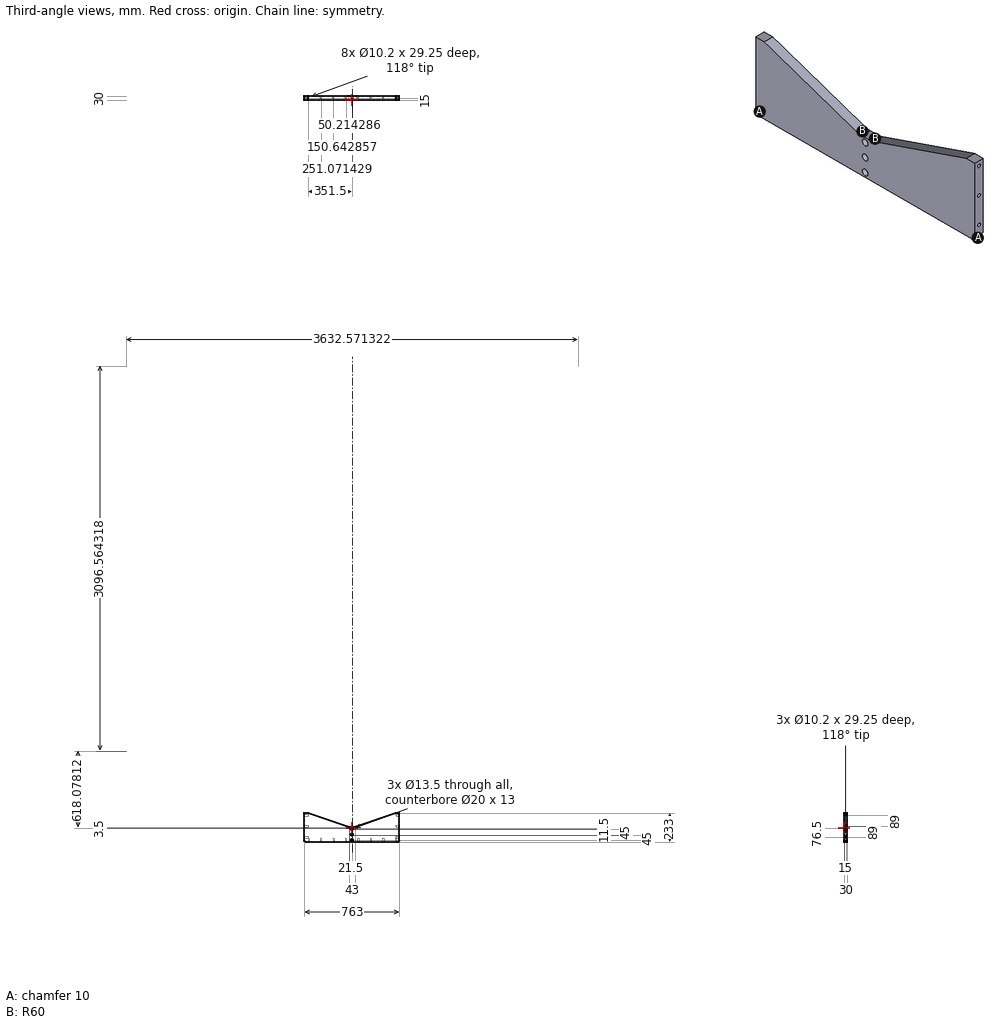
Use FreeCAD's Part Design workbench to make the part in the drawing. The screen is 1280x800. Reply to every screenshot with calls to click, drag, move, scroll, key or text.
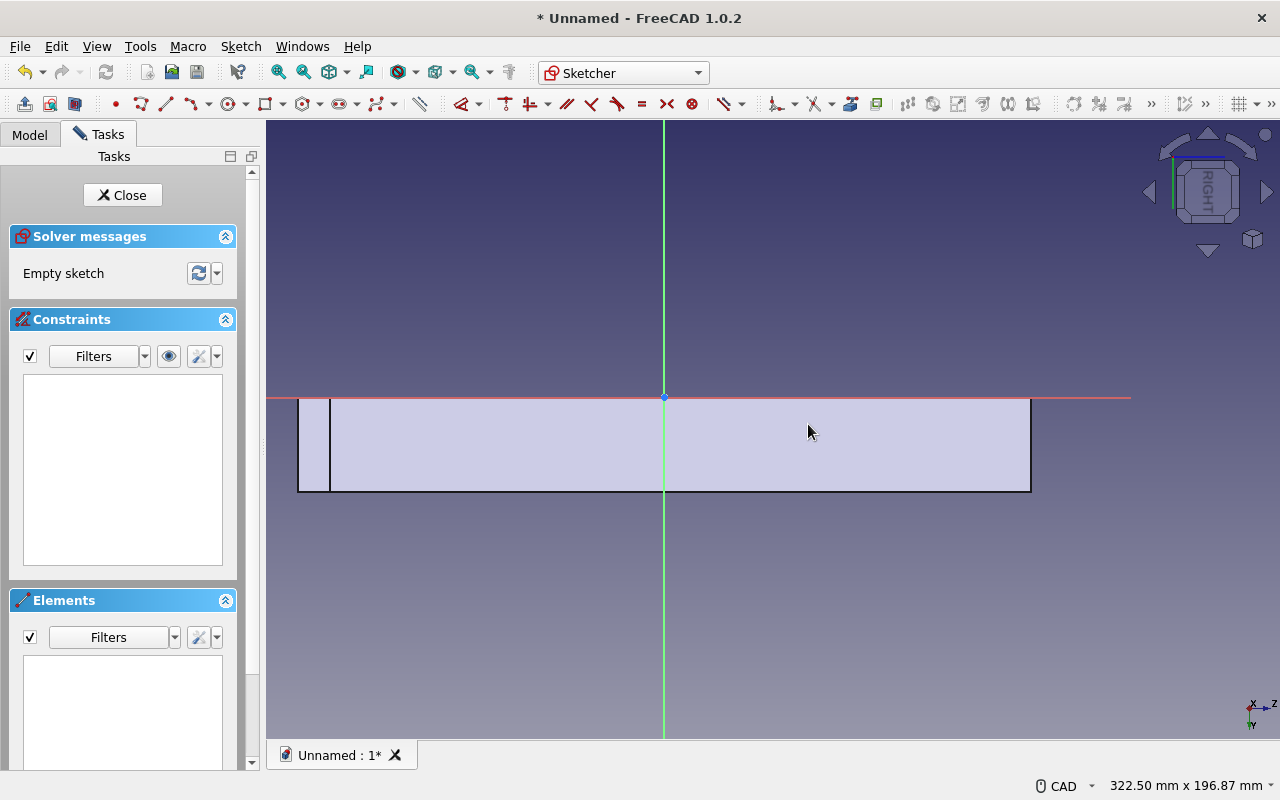
key(g)
key(c)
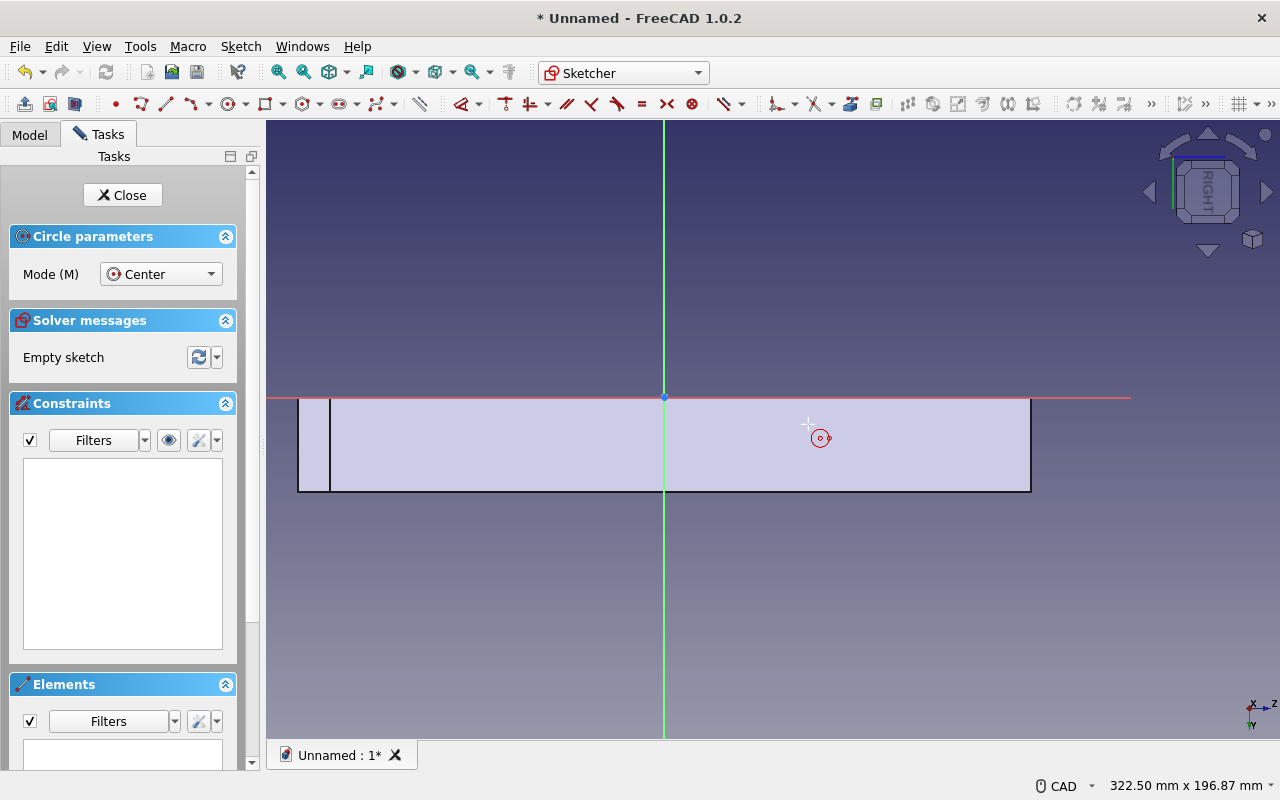
scroll(424, 445, up, 2)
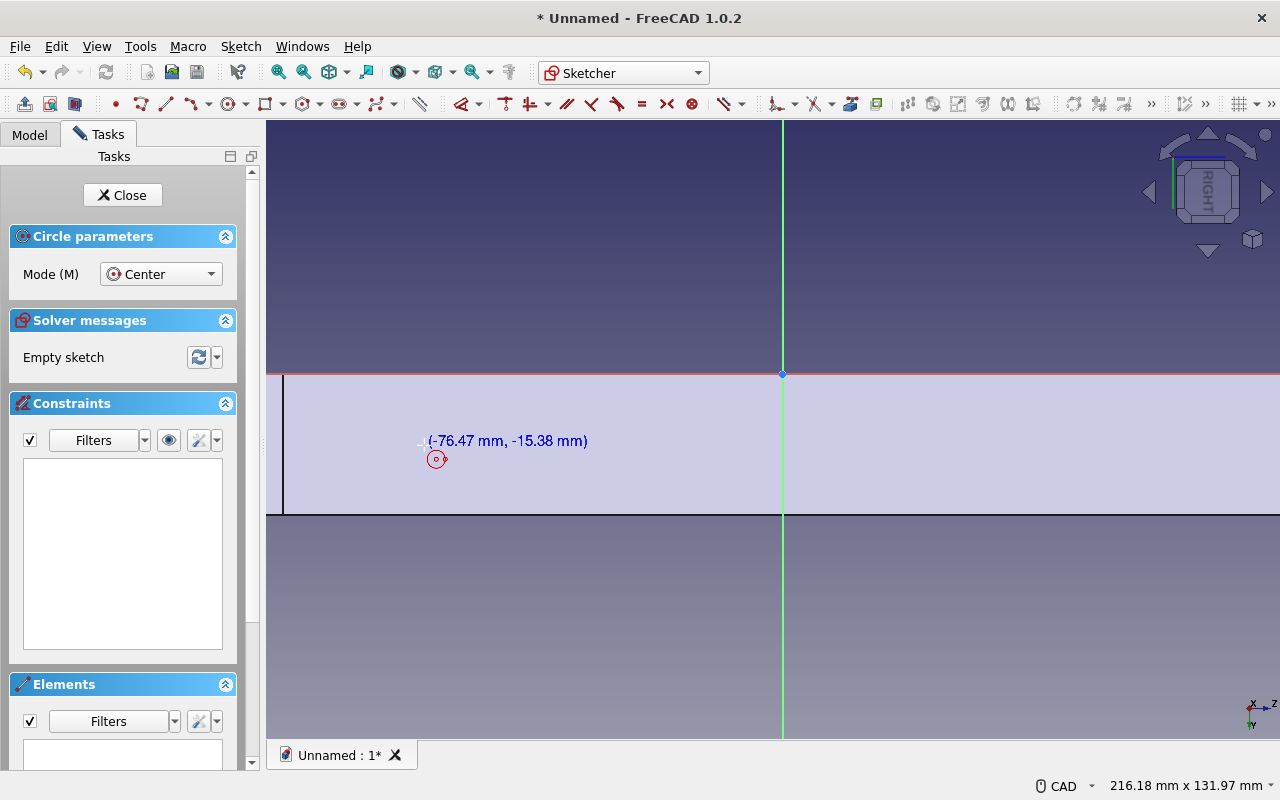
click(424, 444)
click(441, 428)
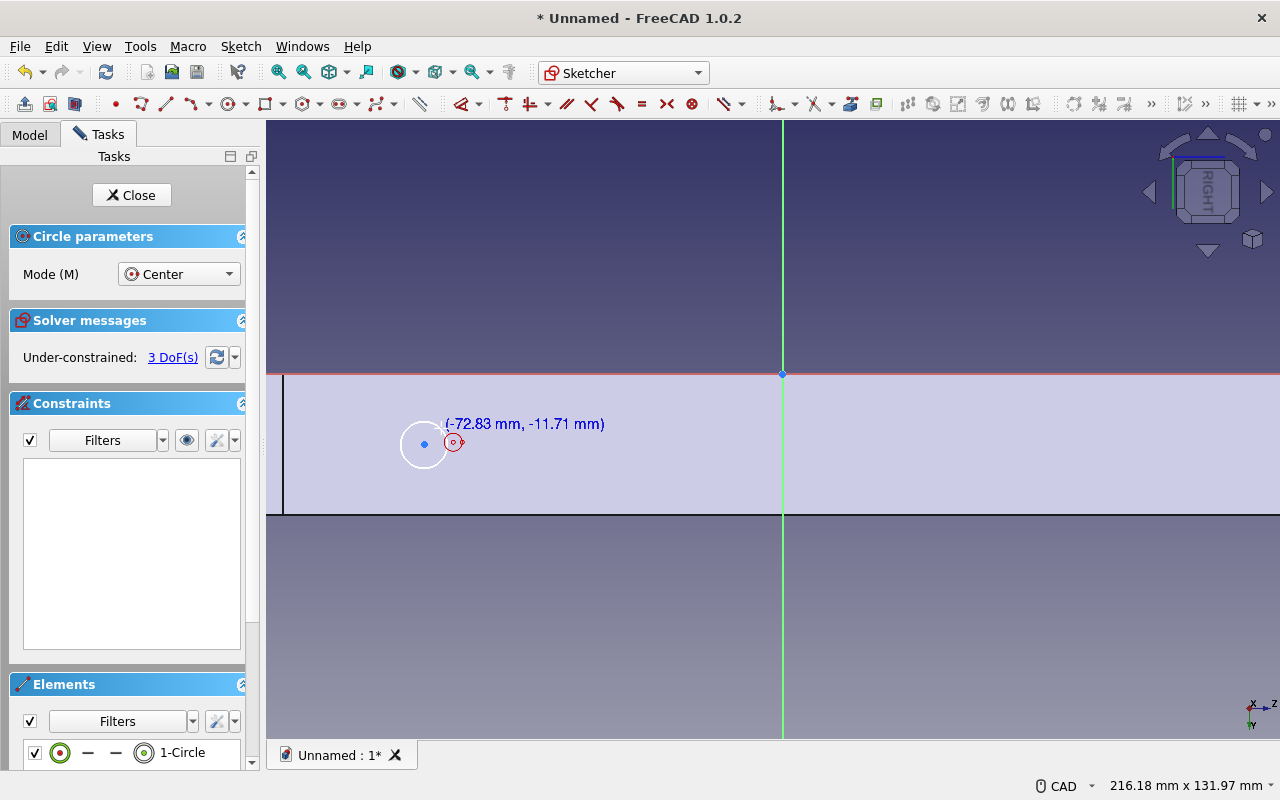
click(841, 444)
click(858, 428)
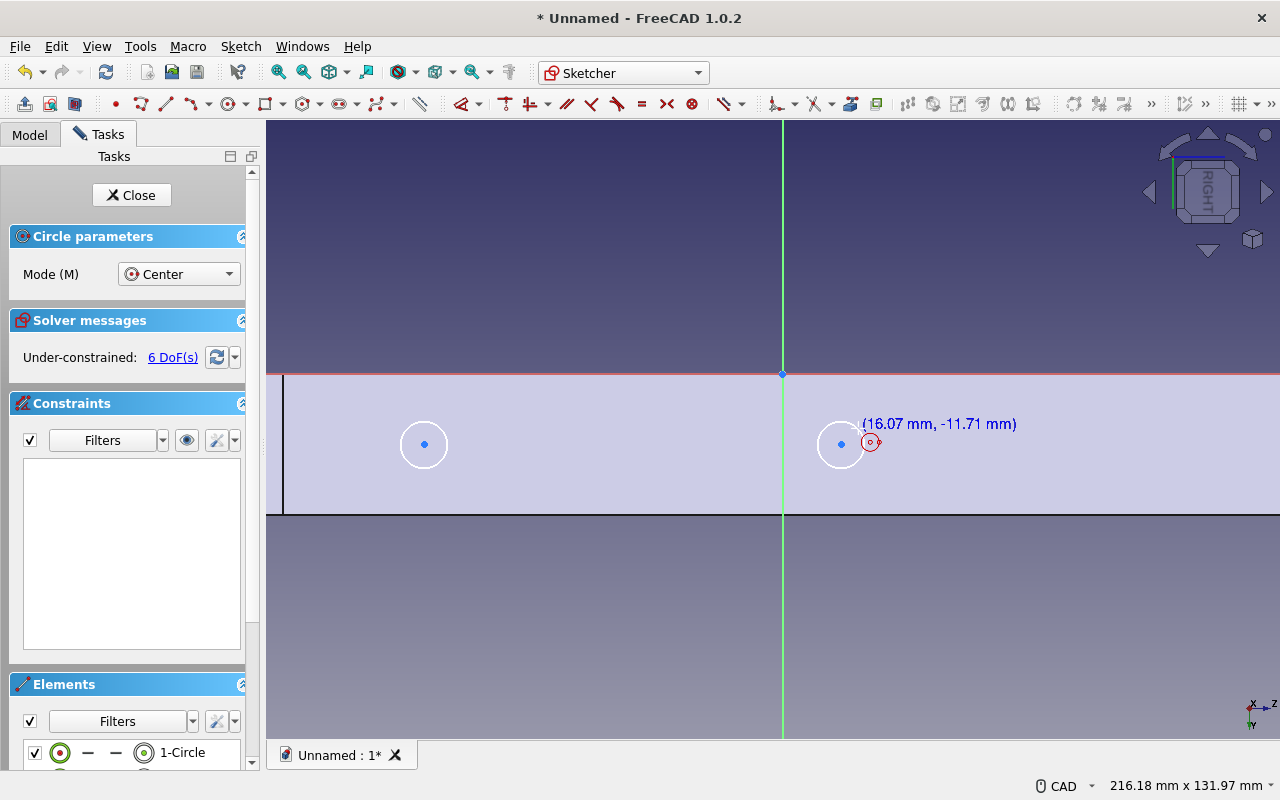
scroll(426, 446, down, 2)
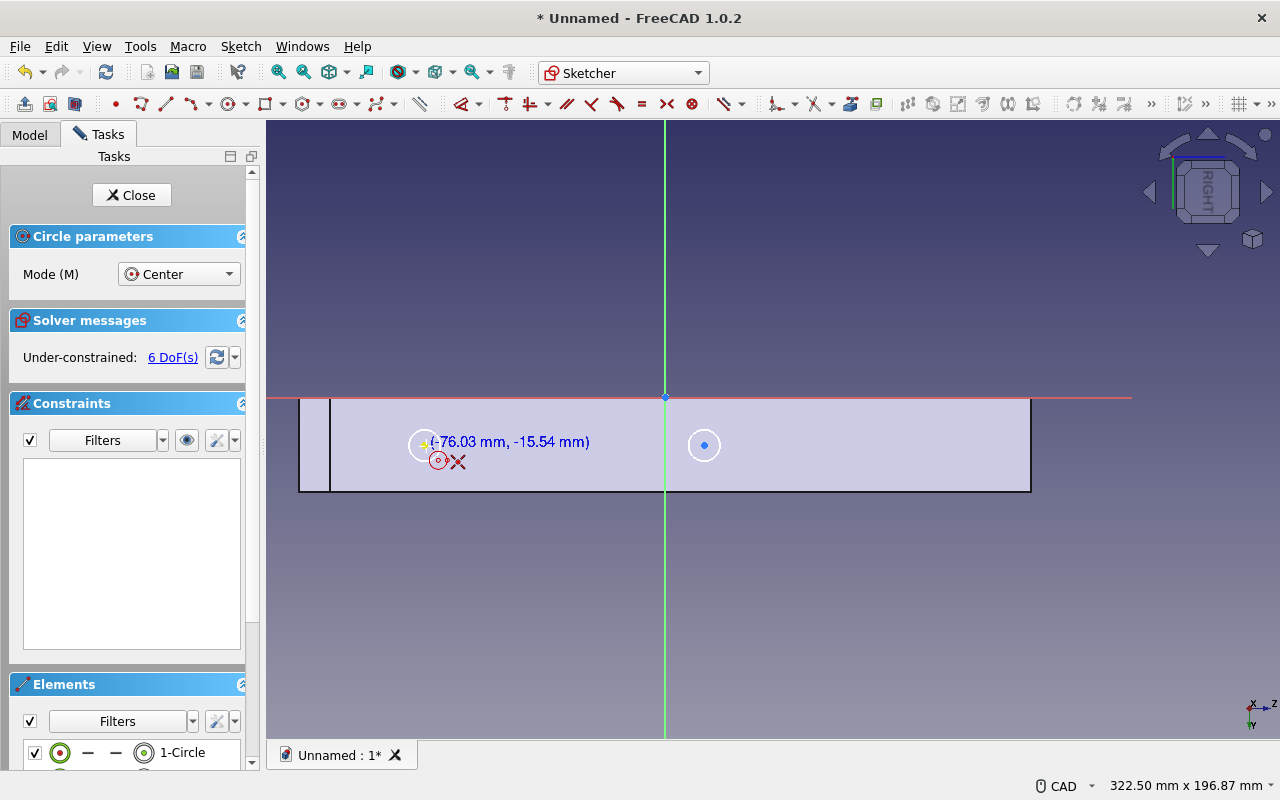
scroll(984, 445, up, 2)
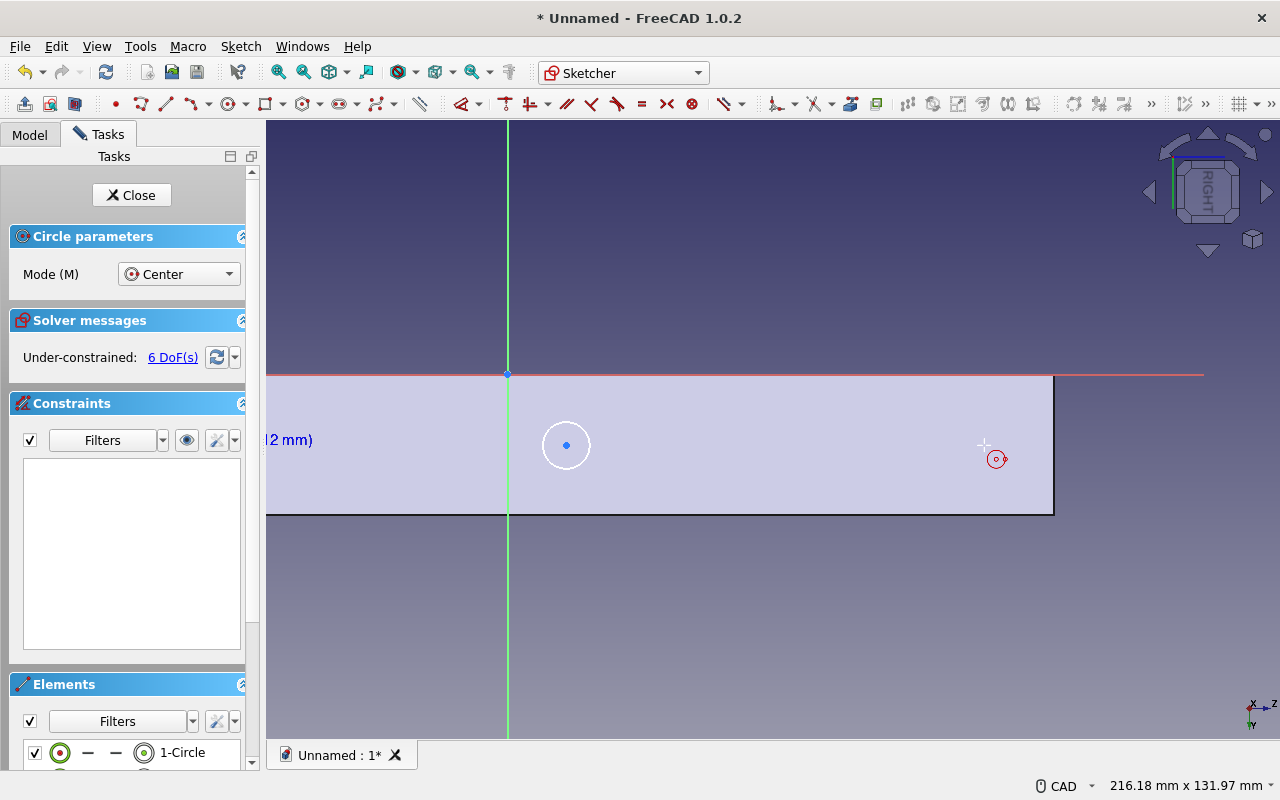
click(984, 445)
click(1001, 428)
key(Escape)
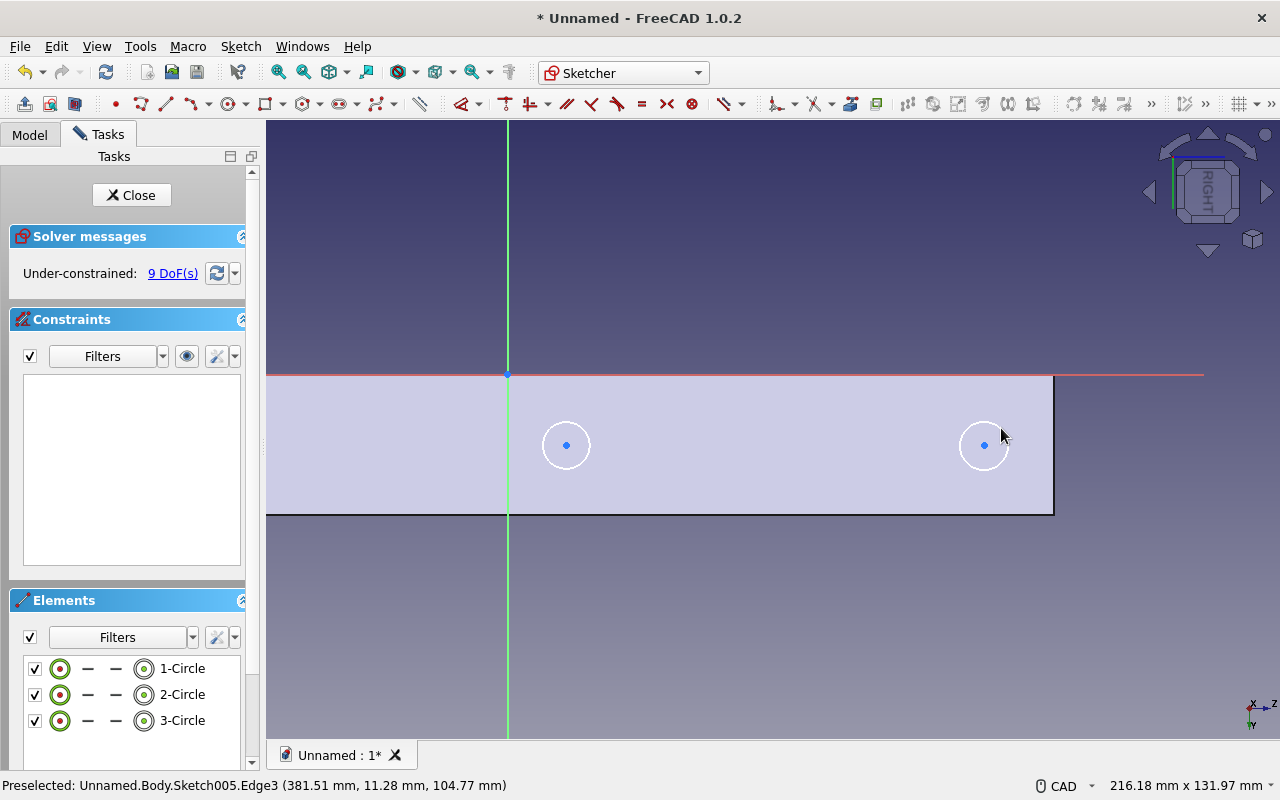
scroll(985, 445, down, 2)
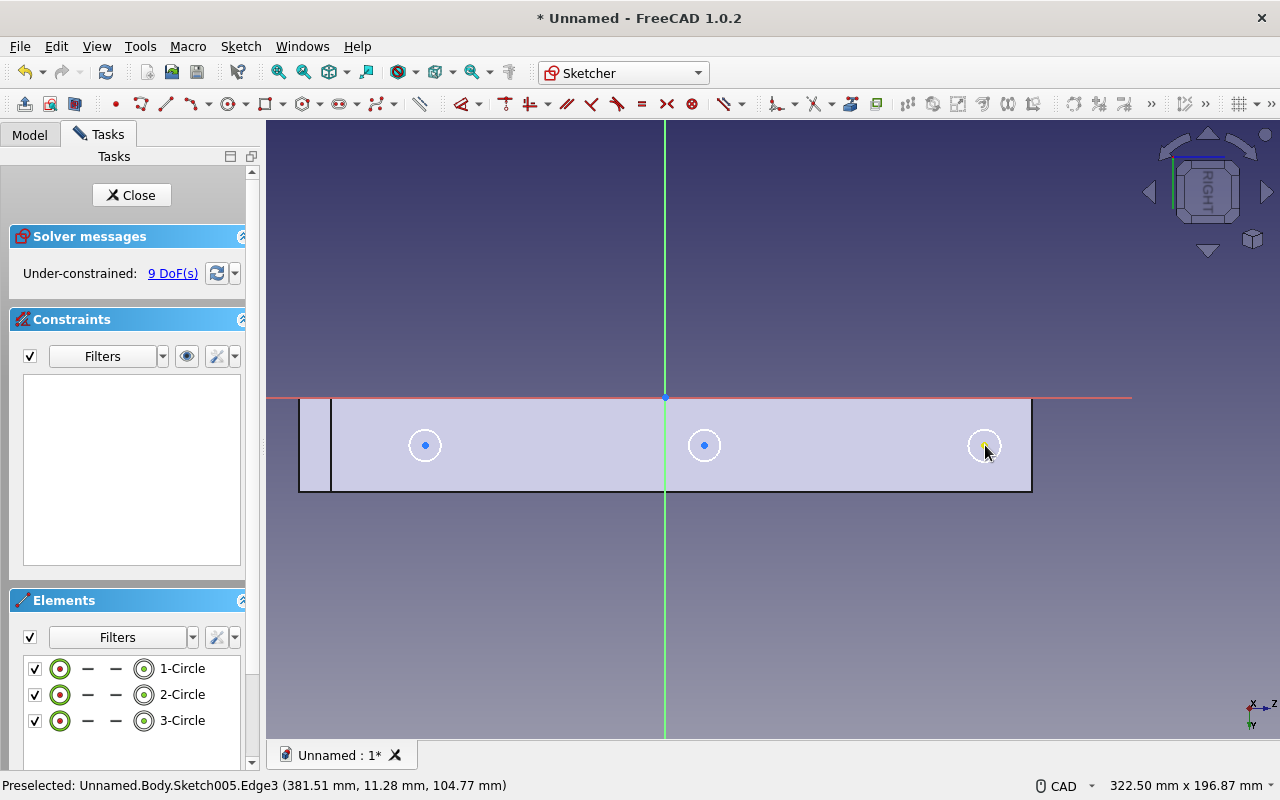
click(436, 434)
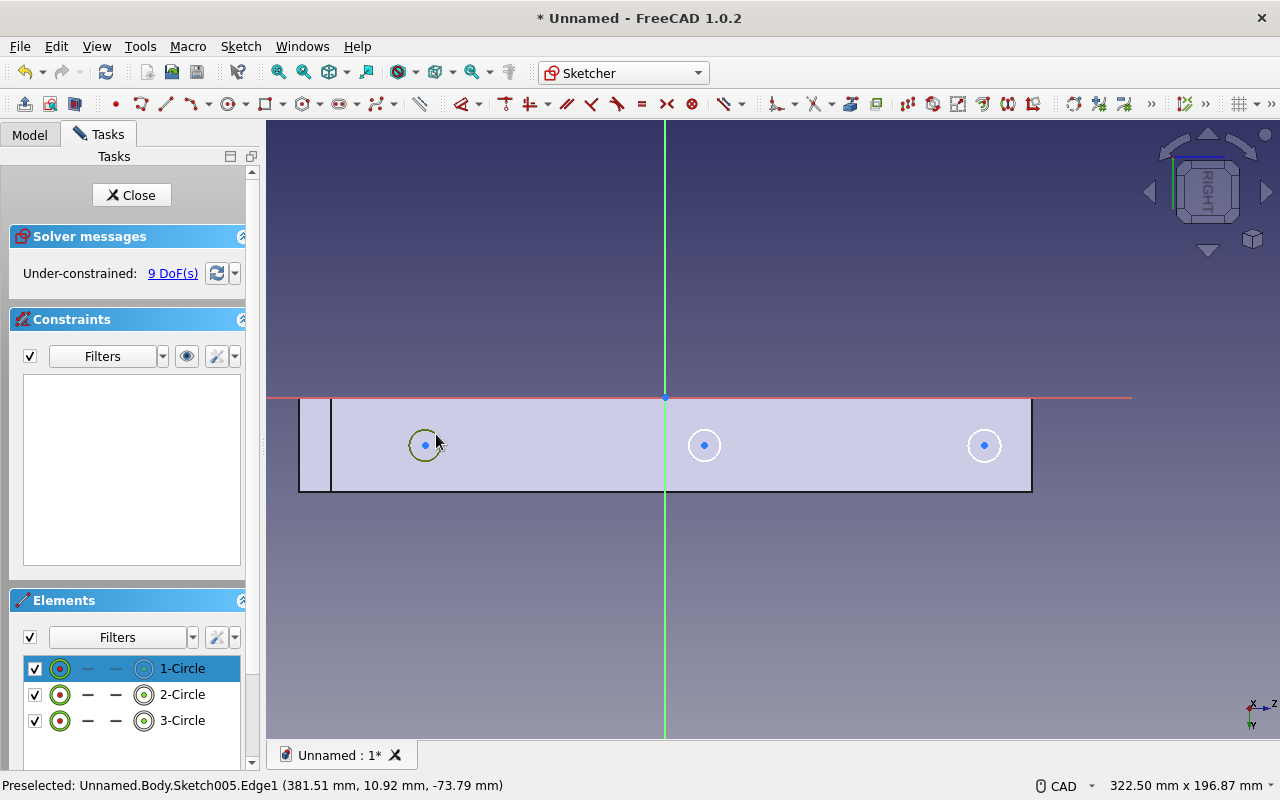
click(716, 434)